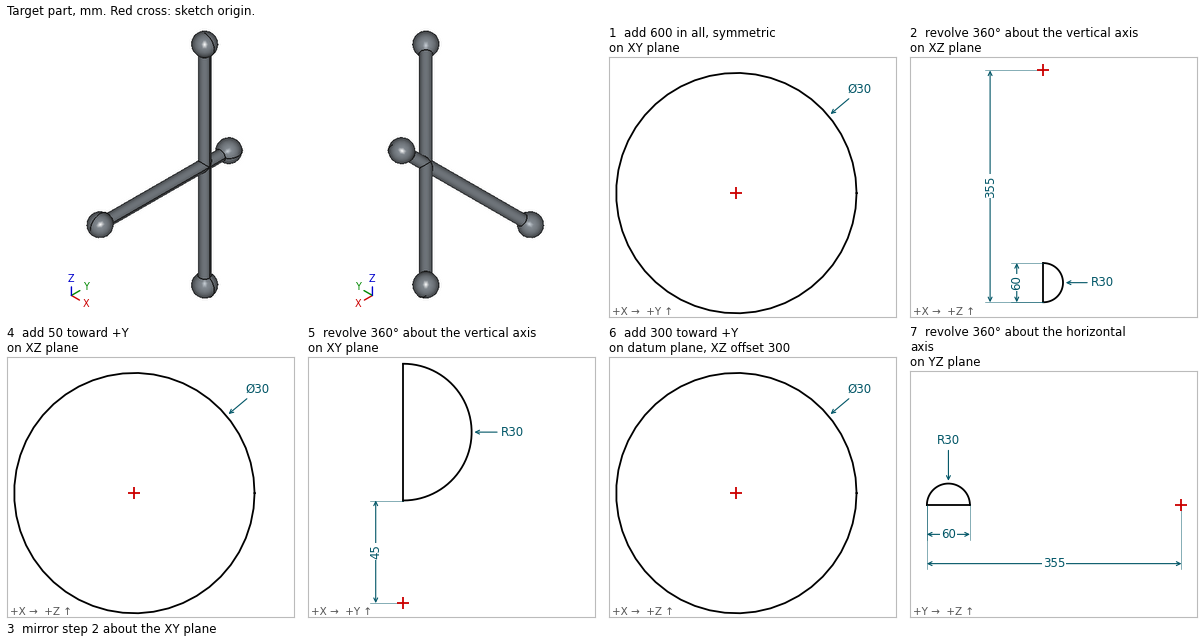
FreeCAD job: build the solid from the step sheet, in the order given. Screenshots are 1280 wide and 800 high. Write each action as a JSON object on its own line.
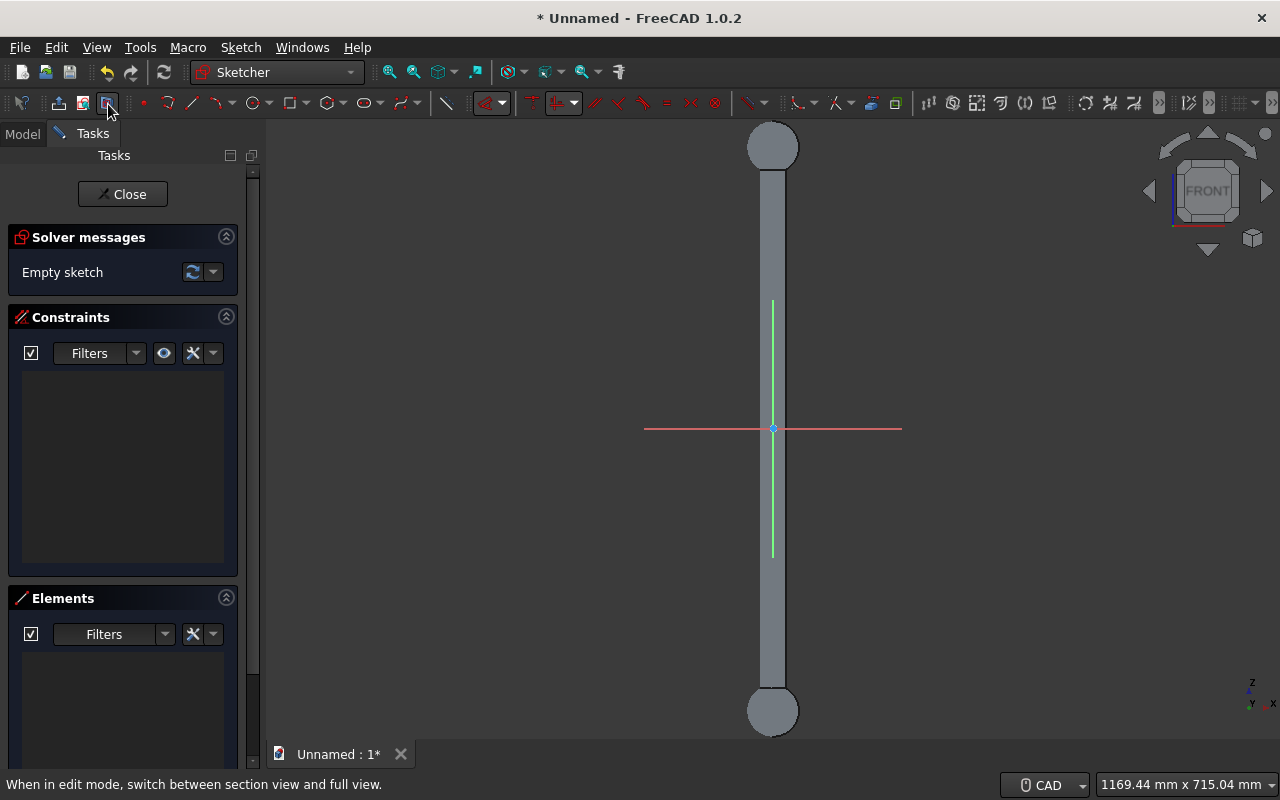
{"action": "scroll", "coordinate": [777, 429], "scroll_direction": "up", "scroll_amount": 14}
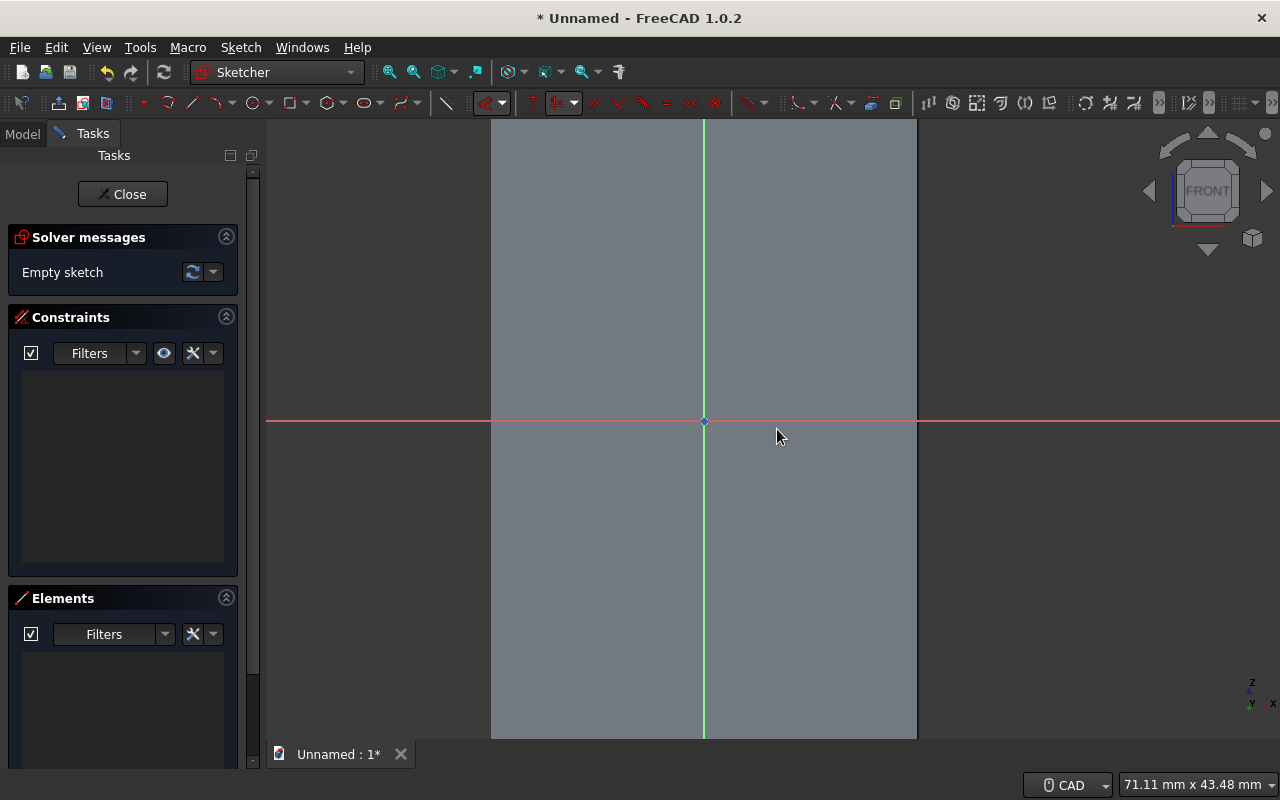
{"action": "key", "text": "g c"}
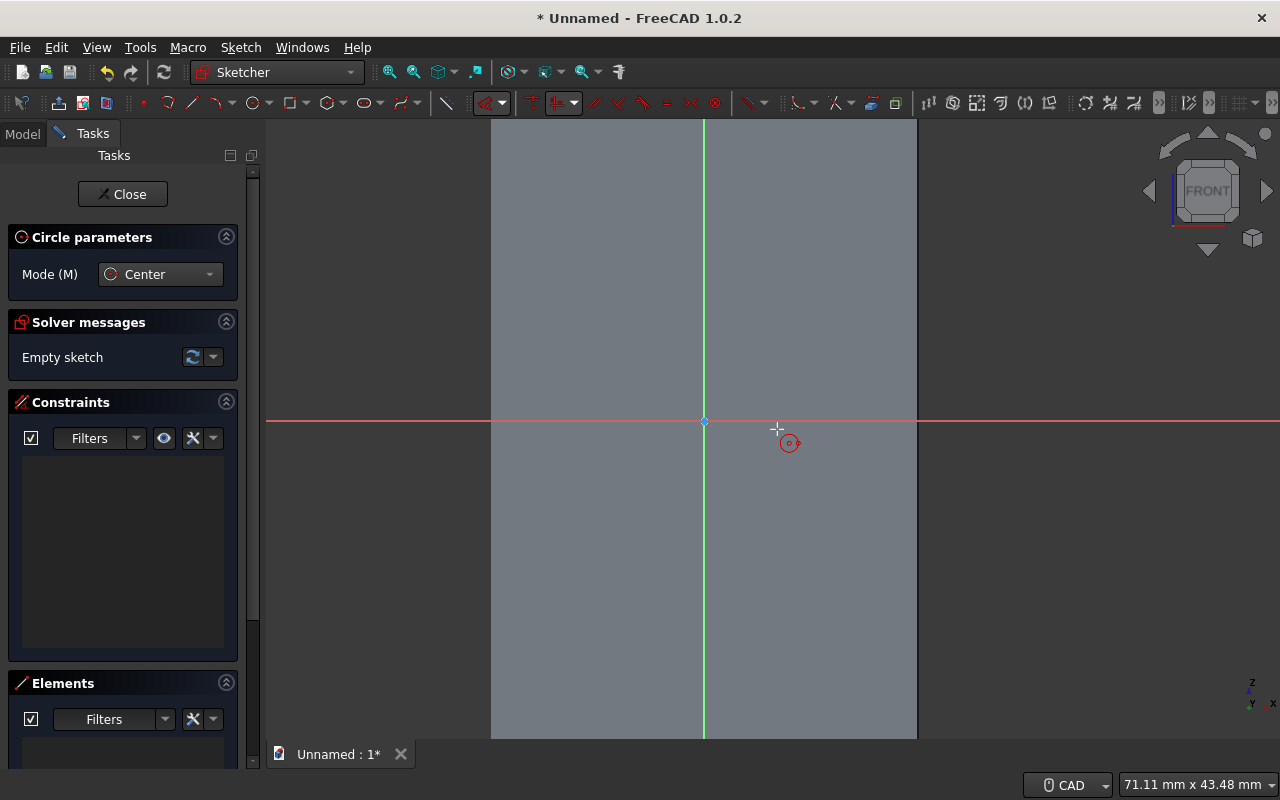
{"action": "left_click", "coordinate": [704, 421]}
{"action": "left_click", "coordinate": [856, 270]}
{"action": "key", "text": "Escape"}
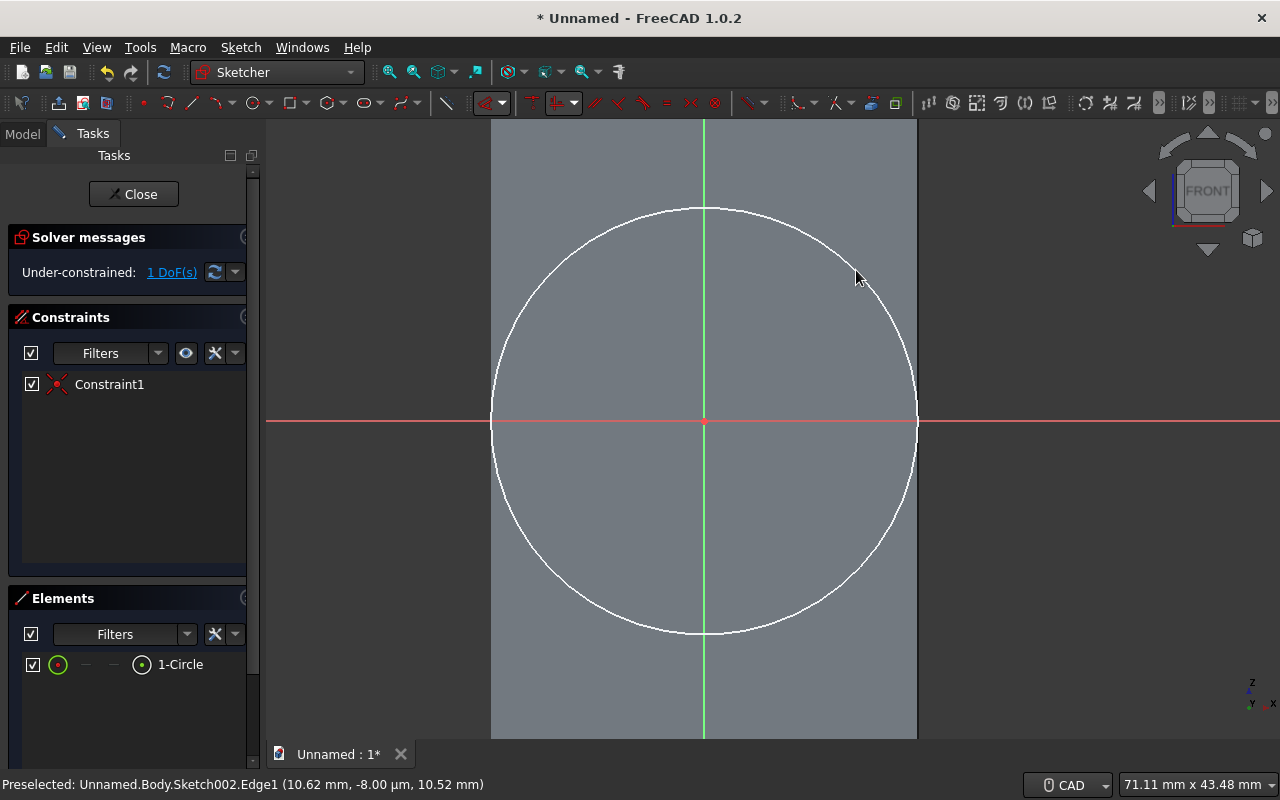
{"action": "left_click", "coordinate": [855, 270]}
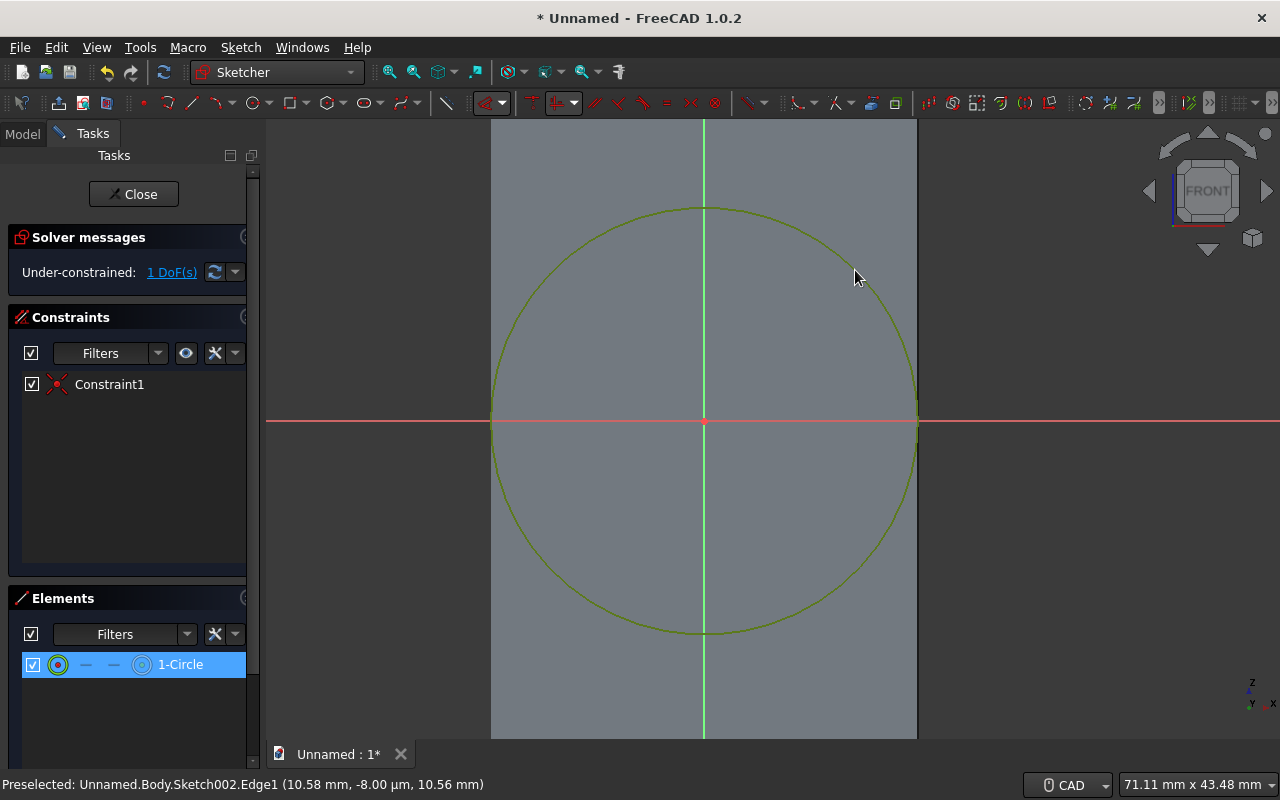
{"action": "key", "text": "k o"}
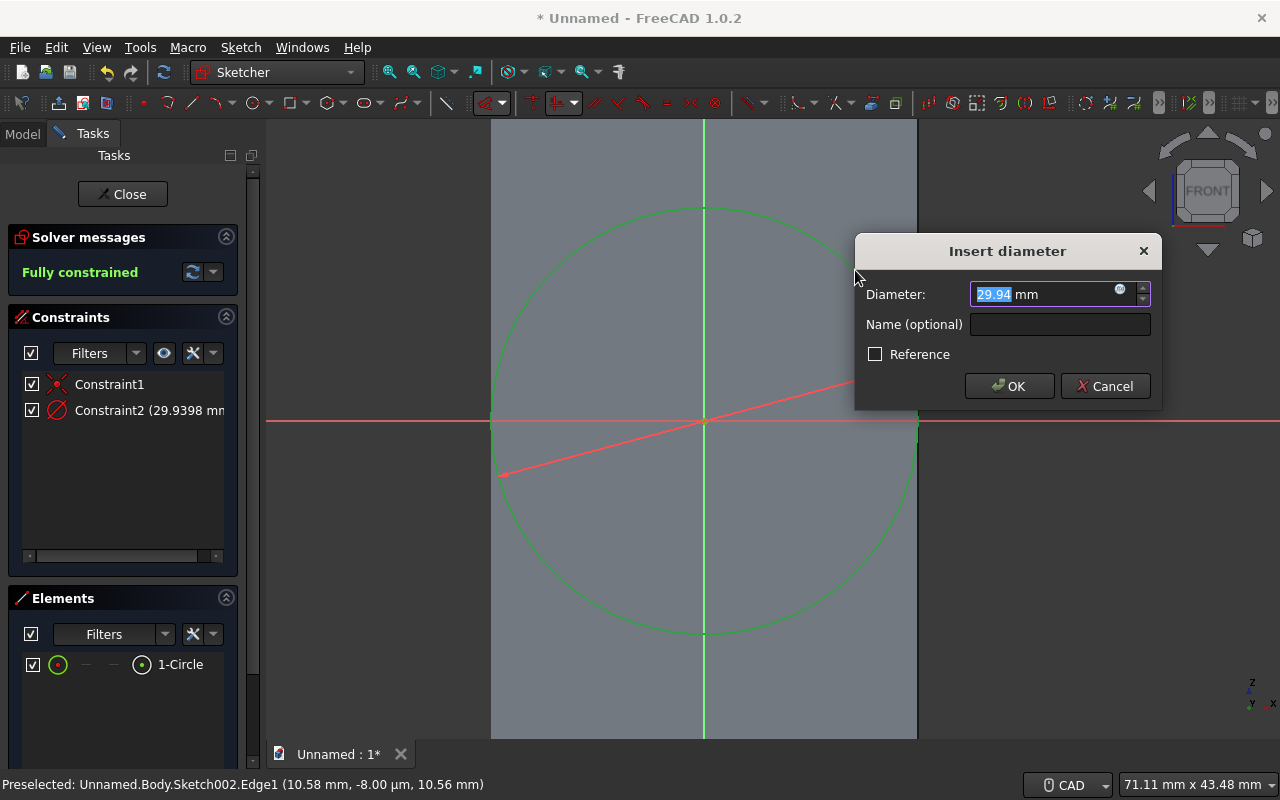
{"action": "type", "text": "30"}
{"action": "key", "text": "Return"}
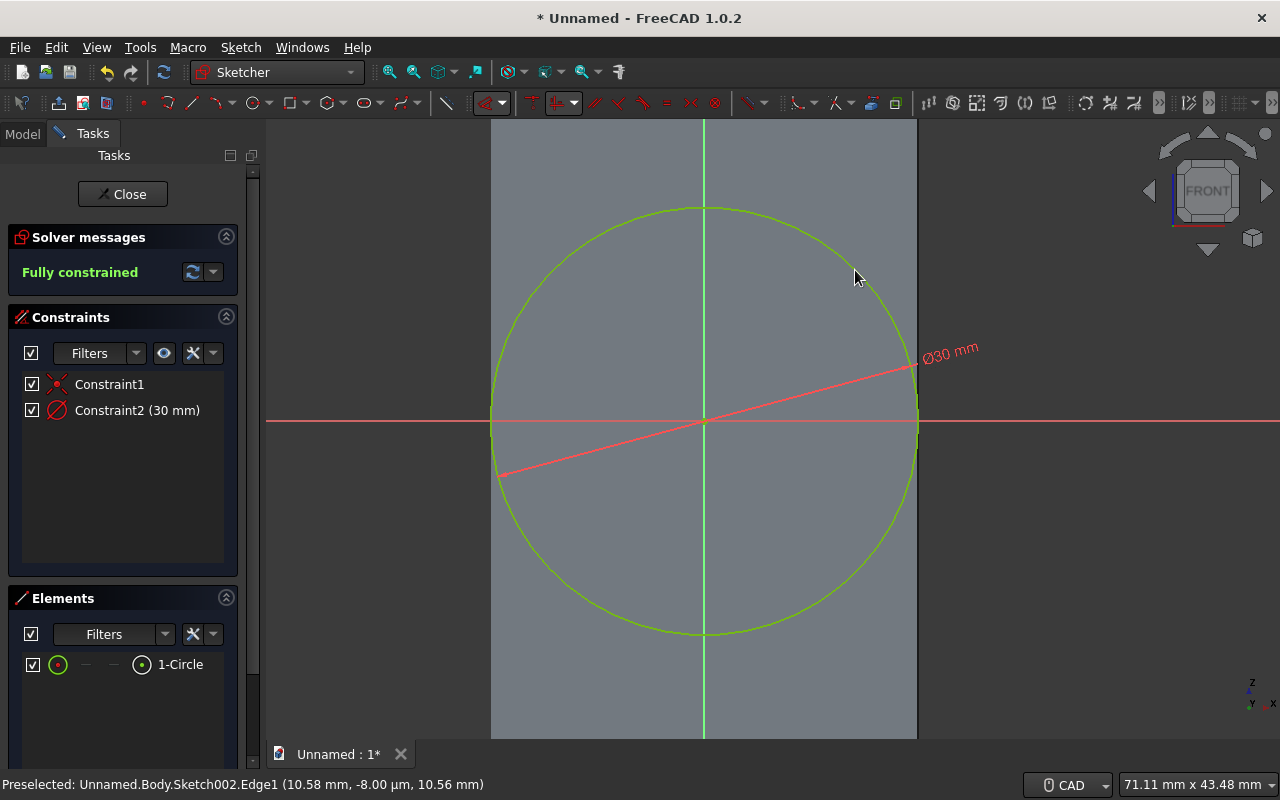
{"action": "left_click", "coordinate": [123, 194]}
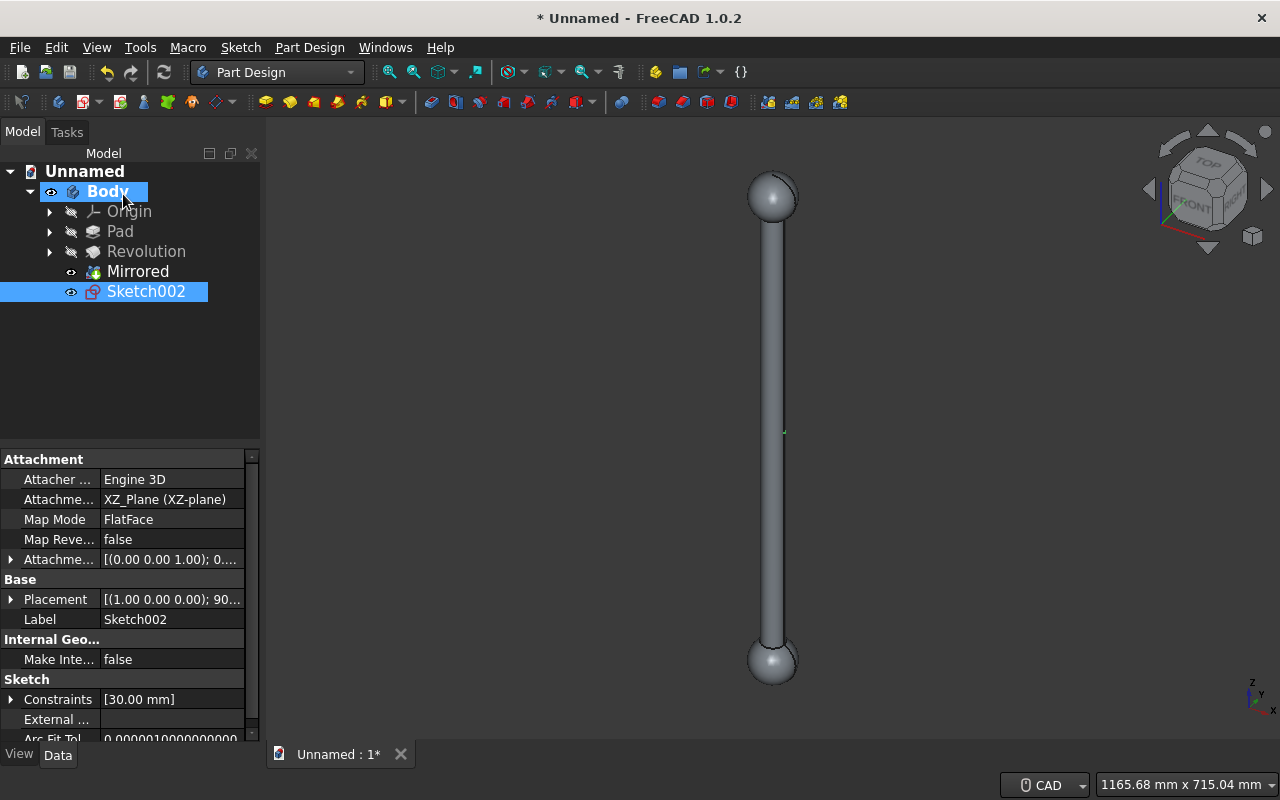
{"action": "left_click", "coordinate": [266, 102]}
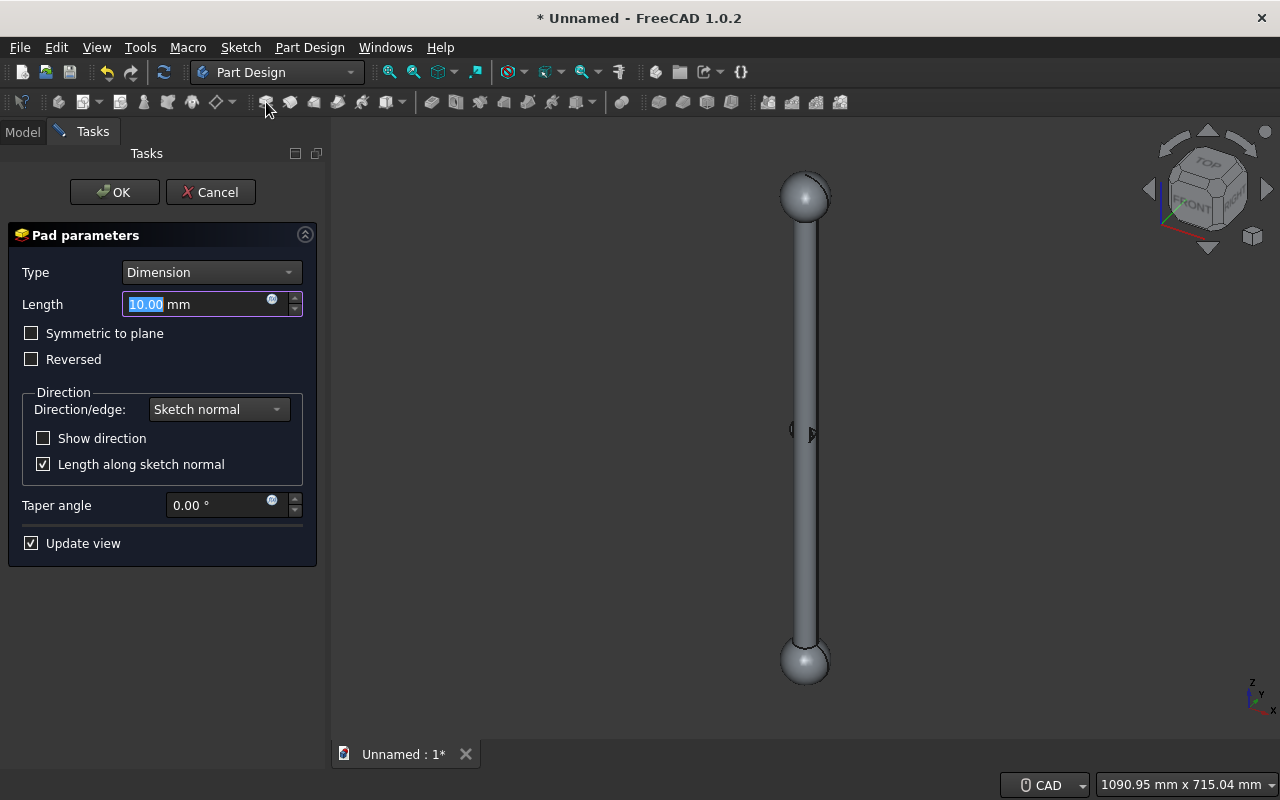
{"action": "type", "text": "50"}
{"action": "key", "text": "Tab"}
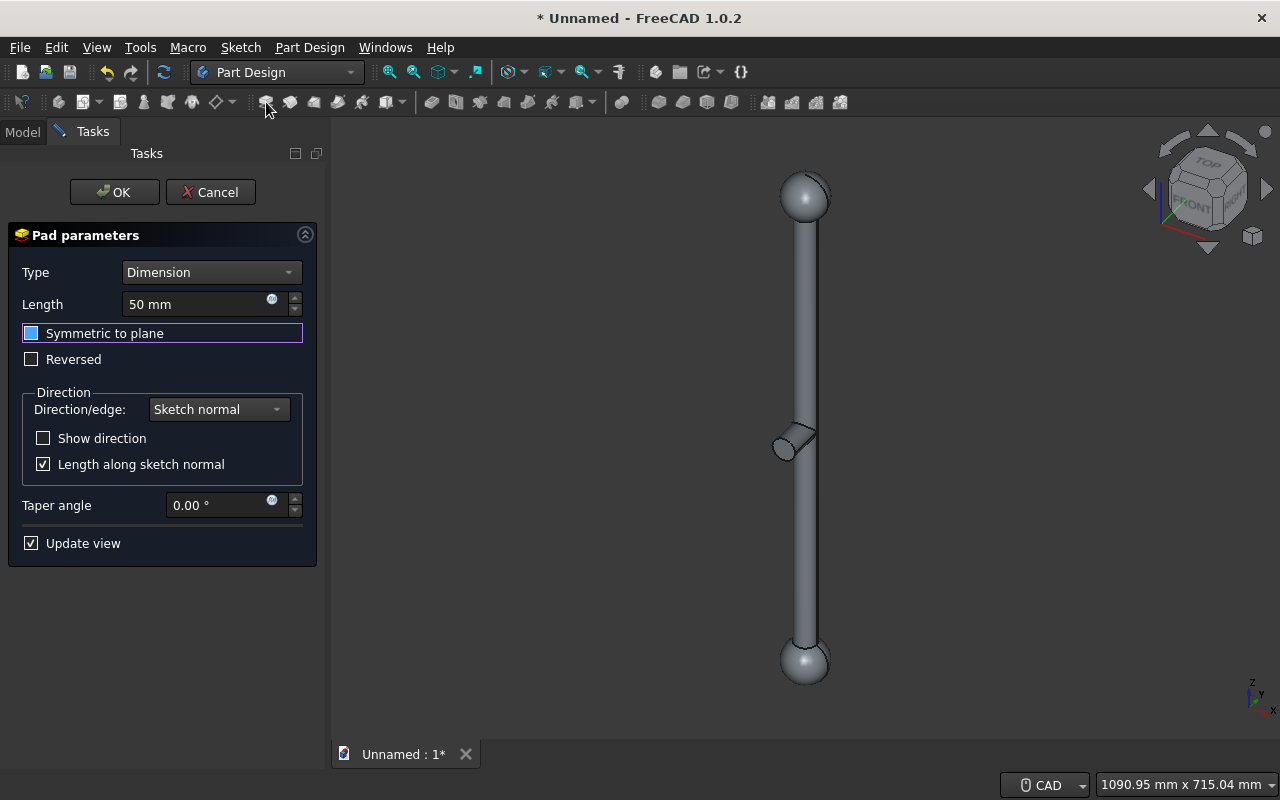
{"action": "left_click", "coordinate": [30, 359]}